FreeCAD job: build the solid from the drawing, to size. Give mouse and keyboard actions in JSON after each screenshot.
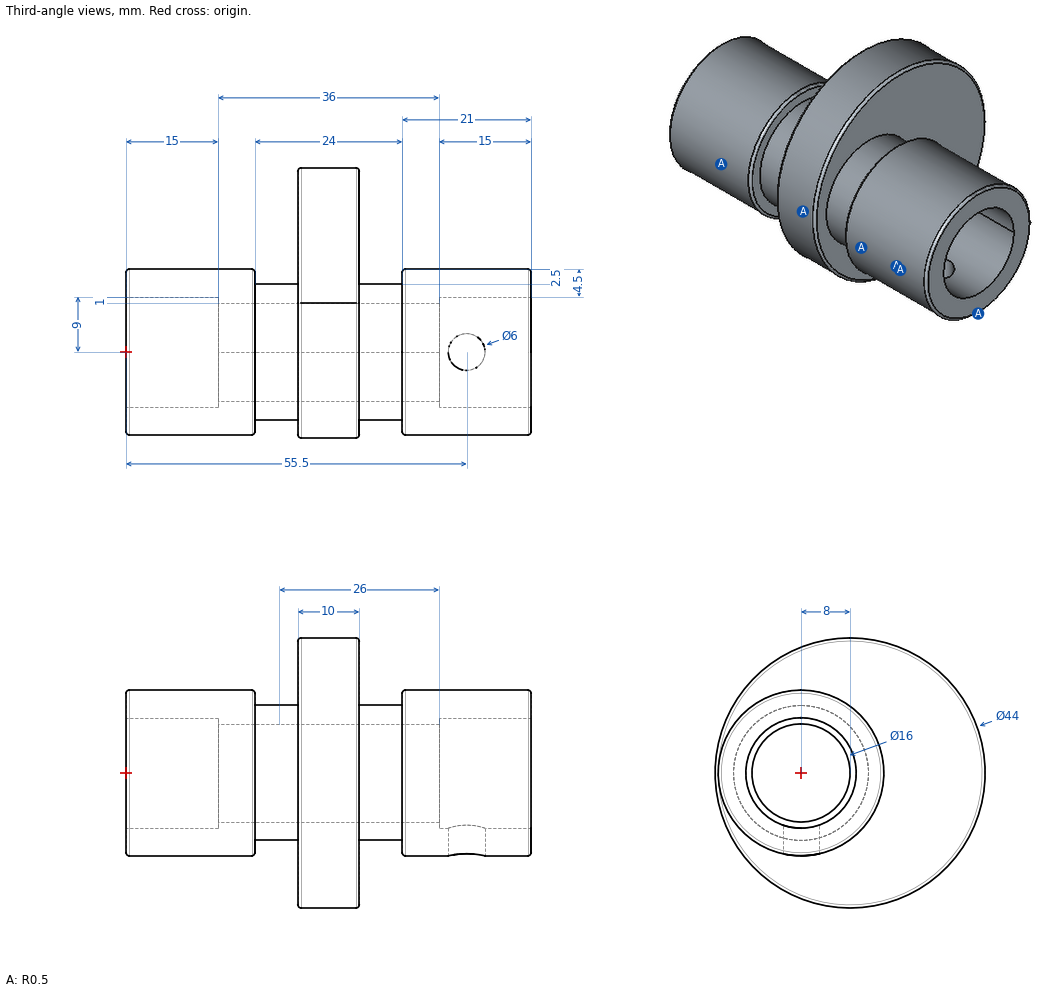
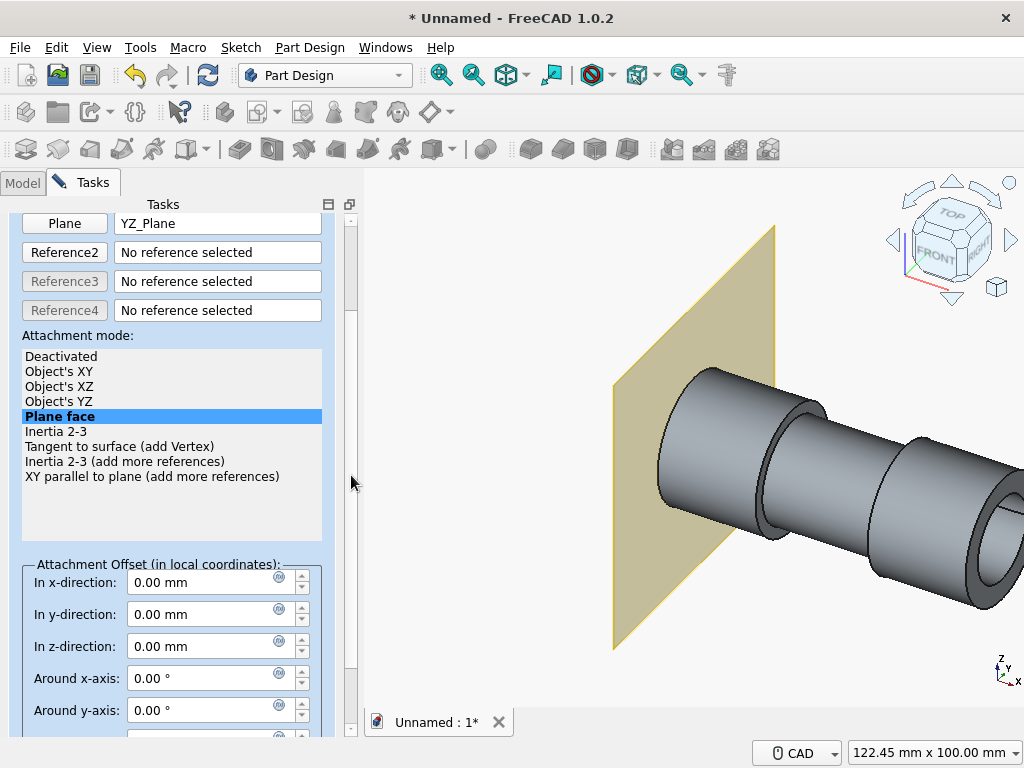
{"action": "triple_click", "coordinate": [210, 646]}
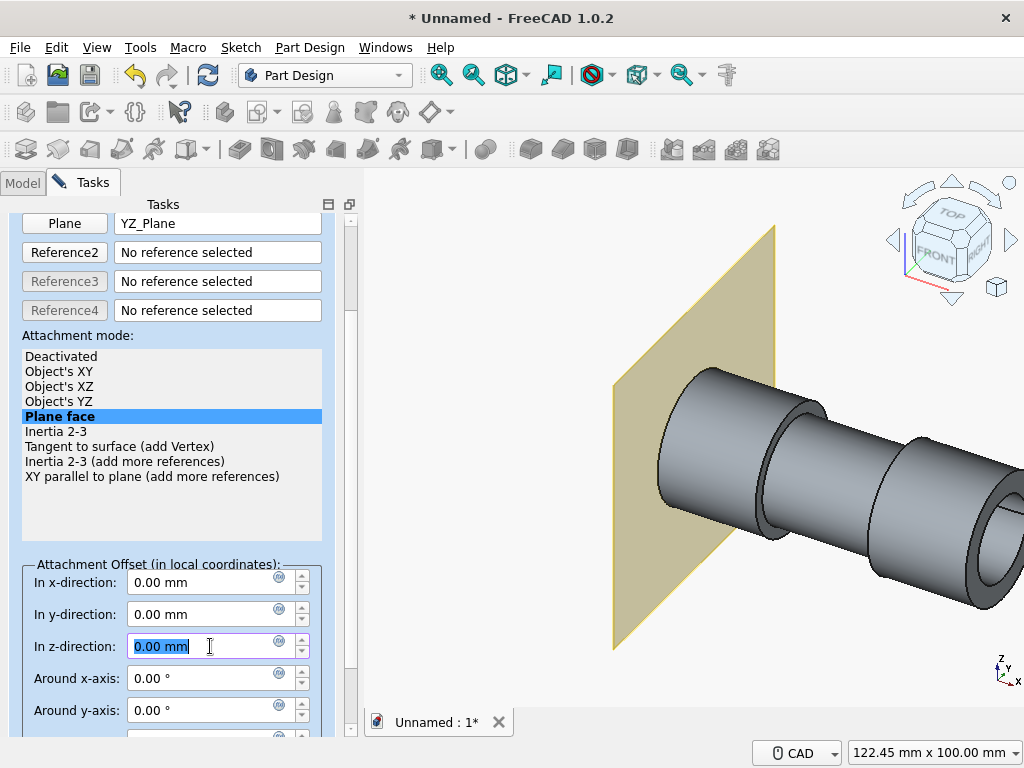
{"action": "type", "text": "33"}
{"action": "key", "text": "Tab"}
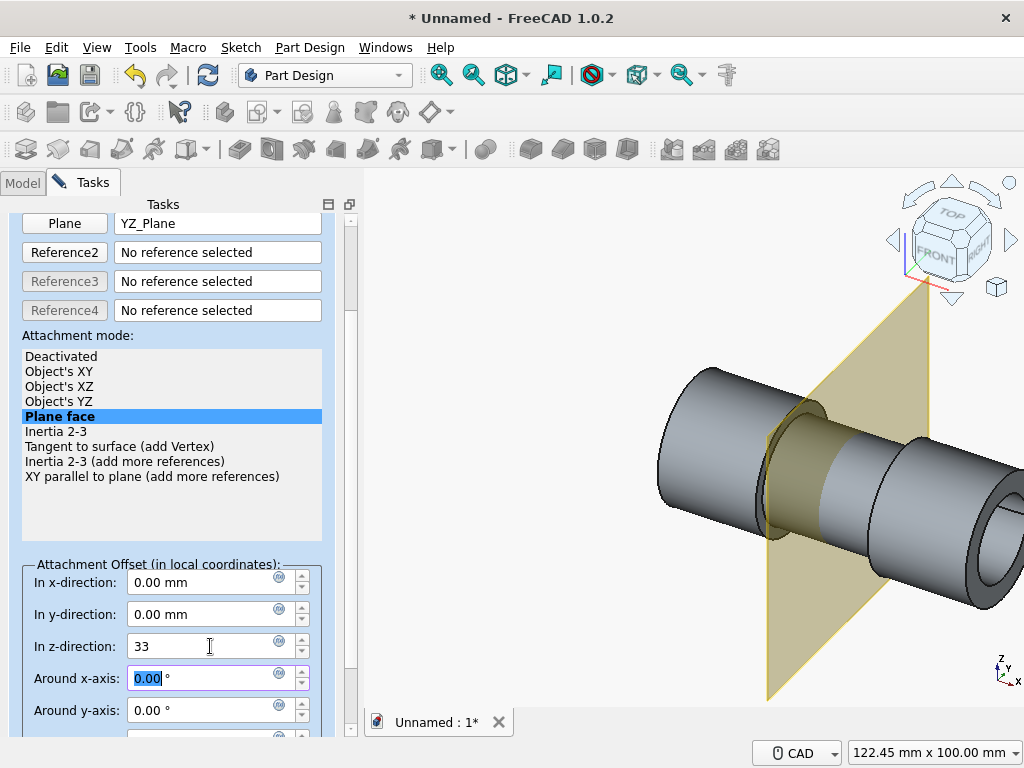
{"action": "scroll", "coordinate": [351, 475], "scroll_direction": "up", "scroll_amount": 3}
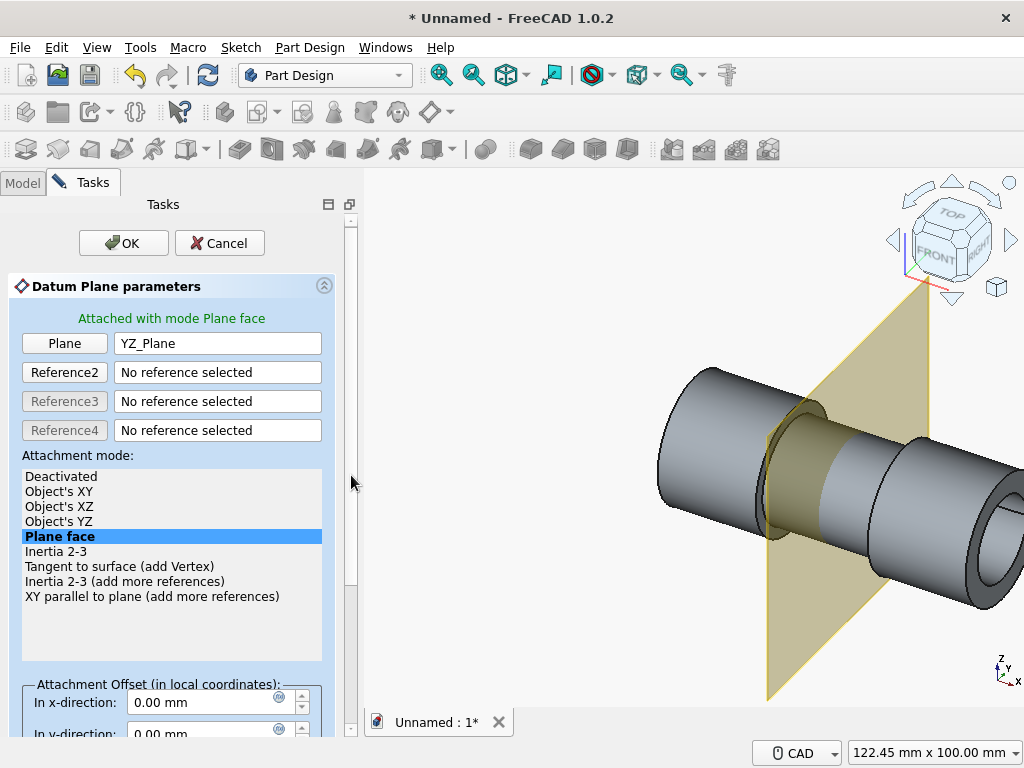
{"action": "left_click", "coordinate": [124, 243]}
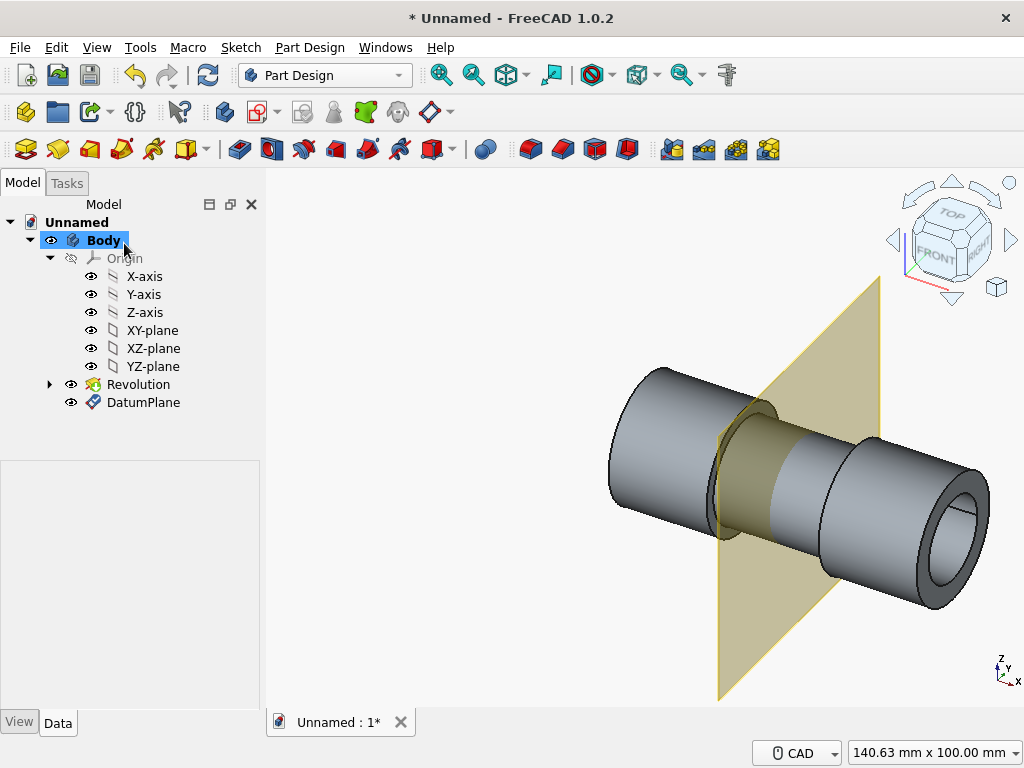
{"action": "left_click", "coordinate": [116, 402]}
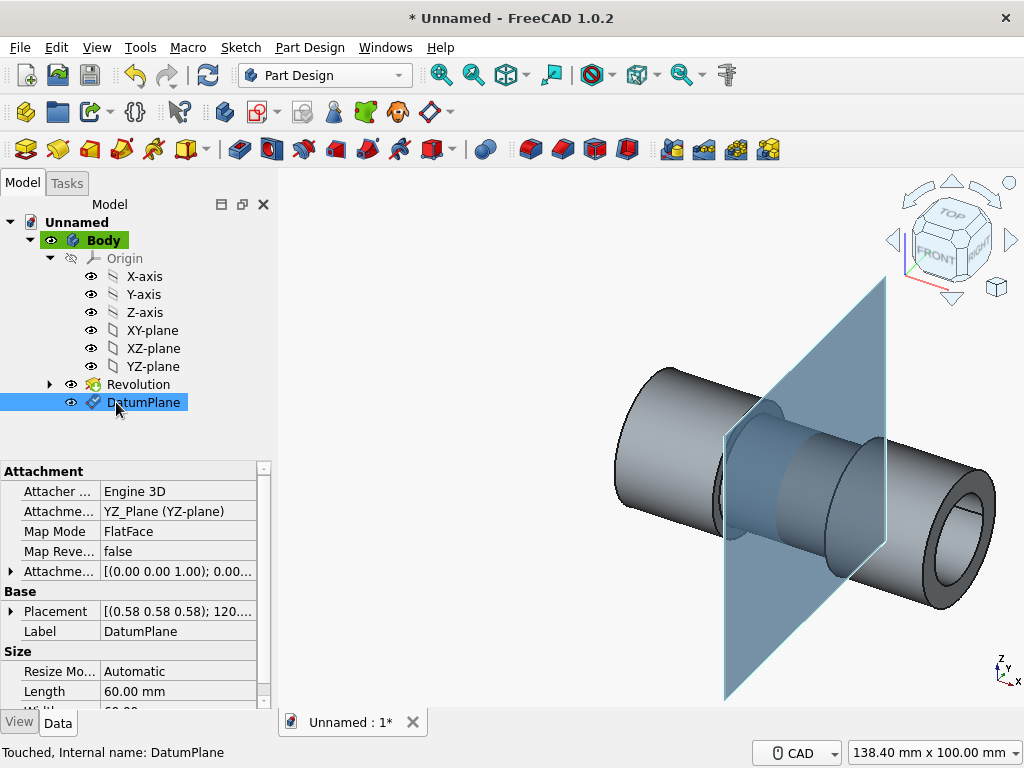
{"action": "left_click", "coordinate": [258, 112]}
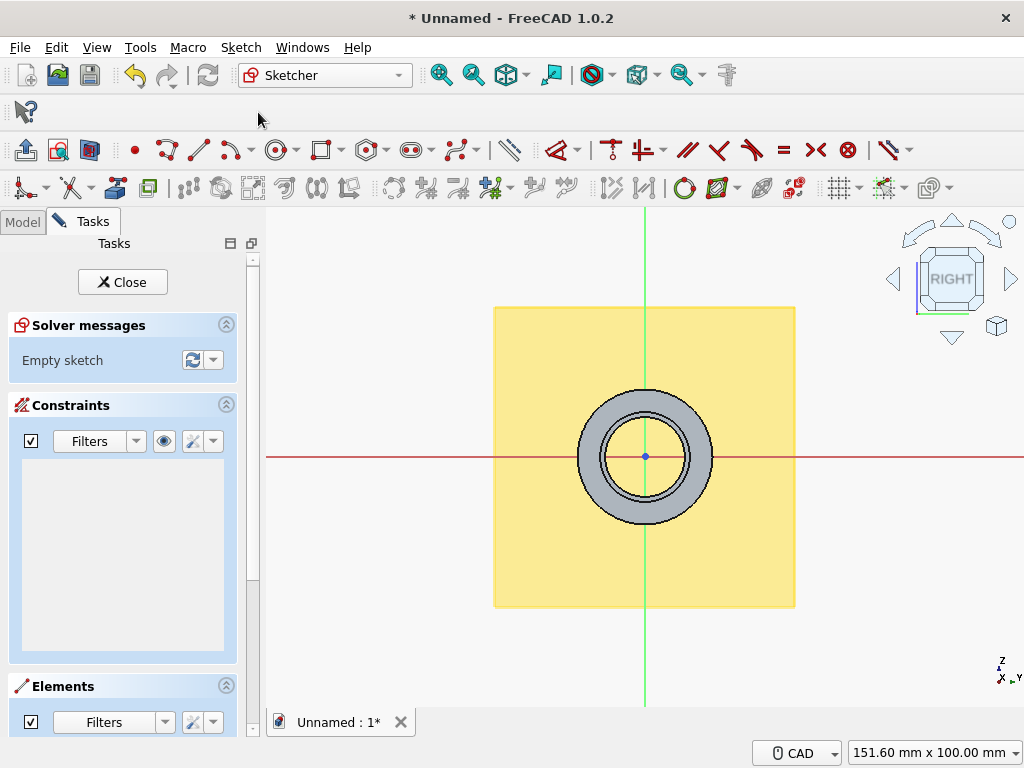
{"action": "left_click", "coordinate": [90, 150]}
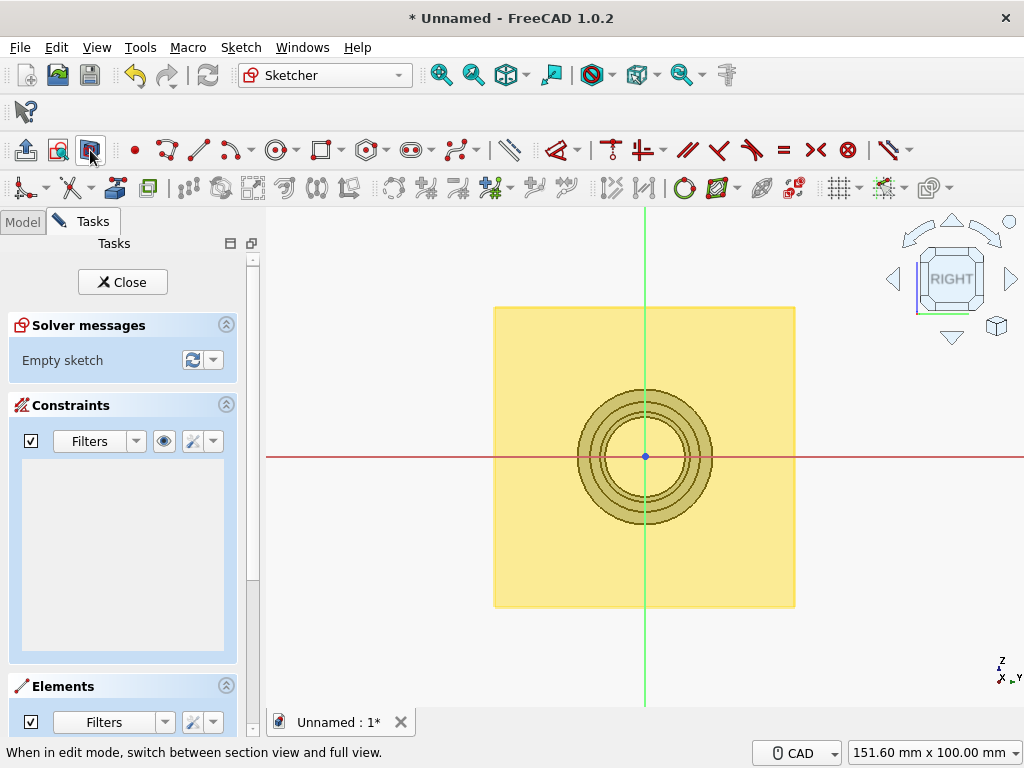
{"action": "scroll", "coordinate": [859, 457], "scroll_direction": "up", "scroll_amount": 2}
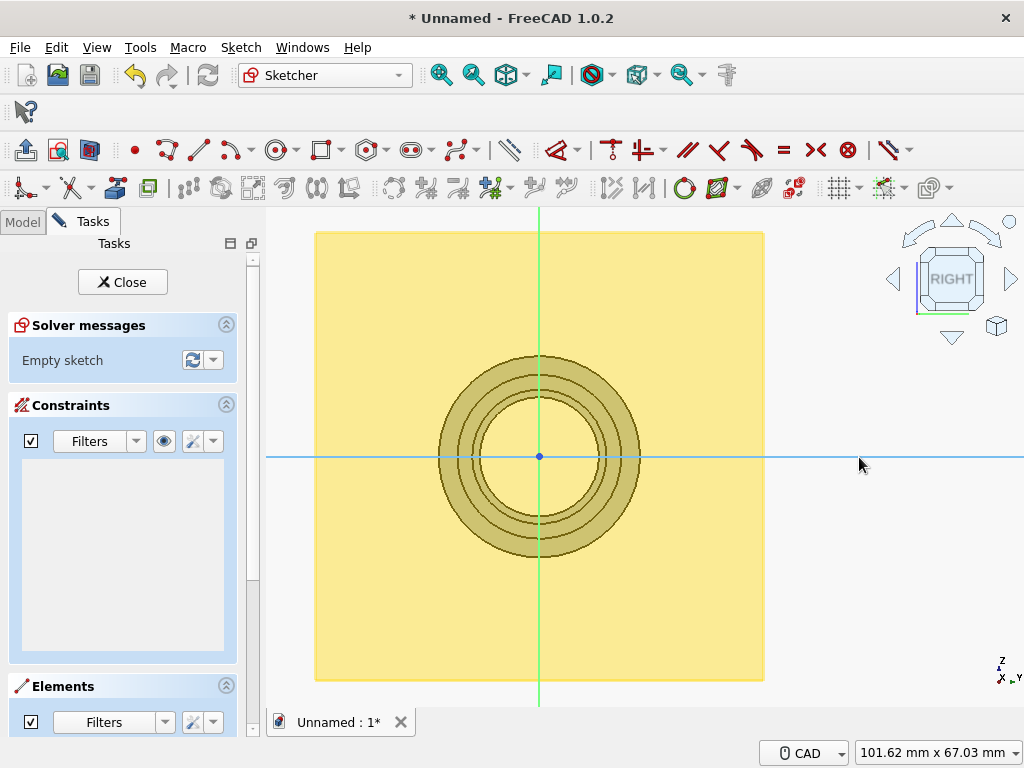
{"action": "left_click", "coordinate": [276, 150]}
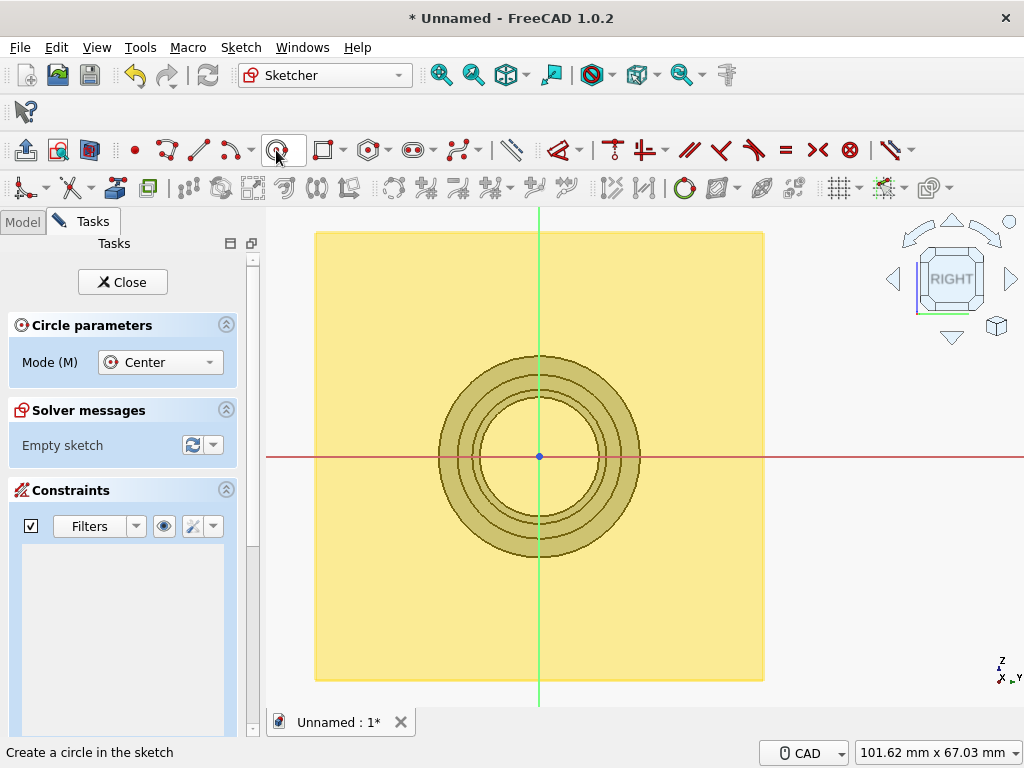
{"action": "left_click", "coordinate": [599, 457]}
{"action": "mouse_move", "coordinate": [715, 341]}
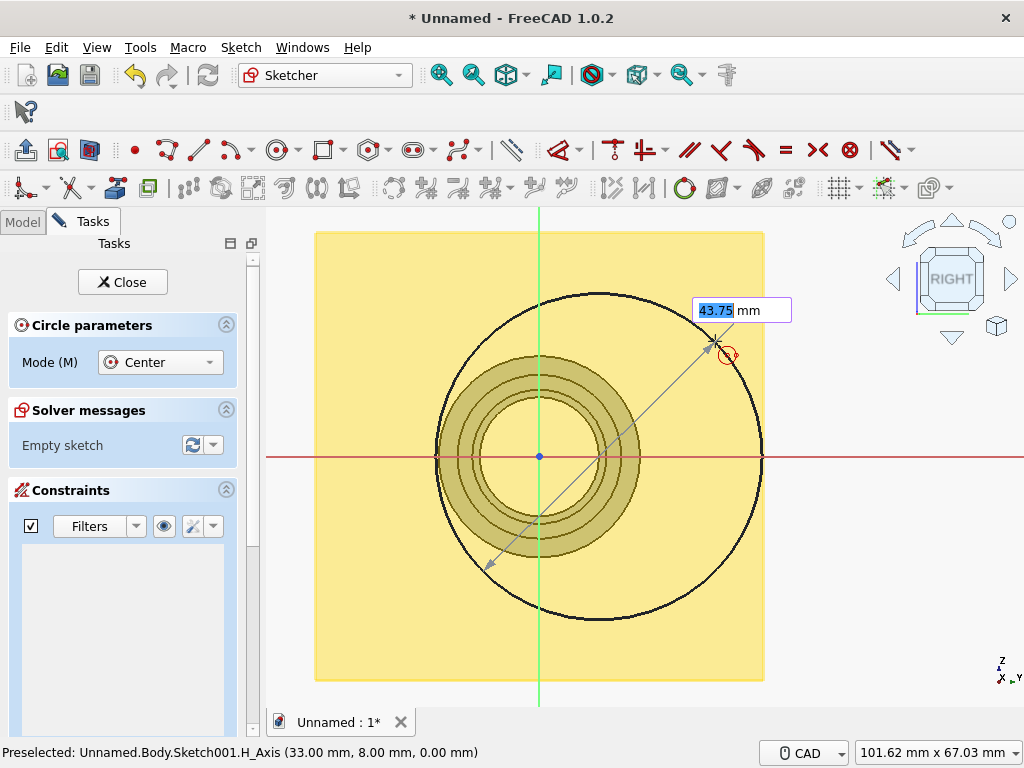
{"action": "type", "text": "44"}
{"action": "key", "text": "Return"}
{"action": "key", "text": "Escape"}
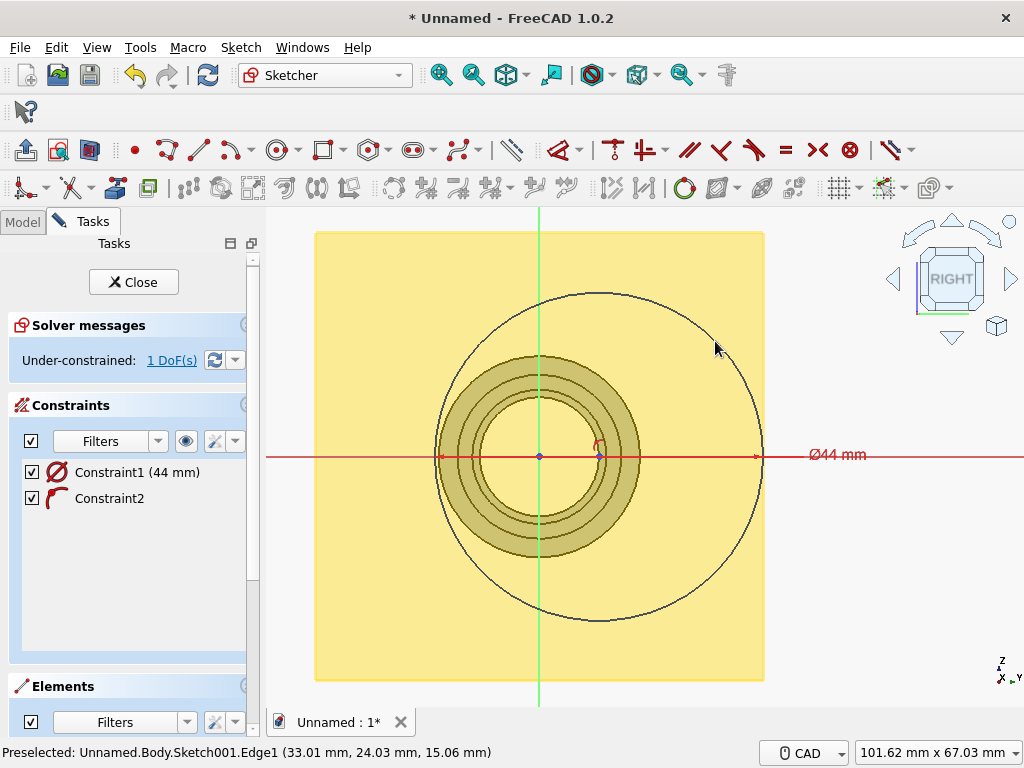
{"action": "left_click", "coordinate": [558, 150]}